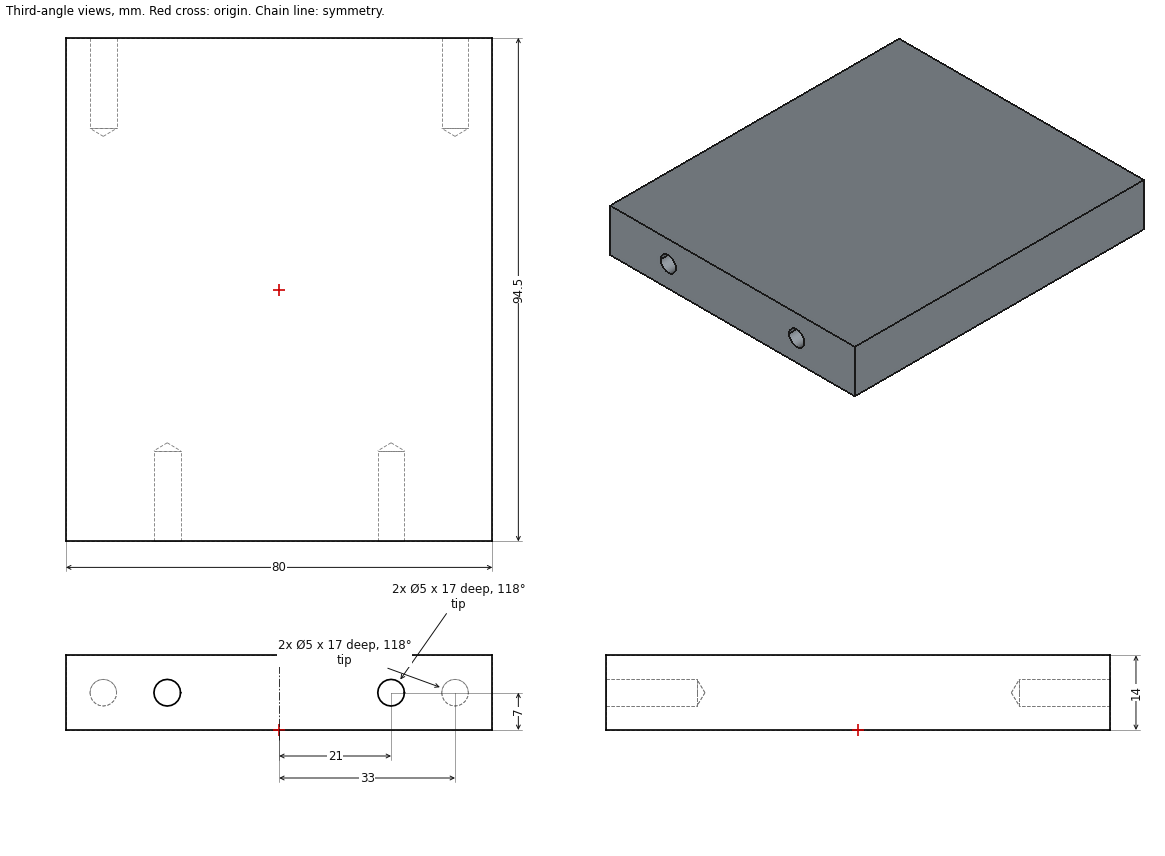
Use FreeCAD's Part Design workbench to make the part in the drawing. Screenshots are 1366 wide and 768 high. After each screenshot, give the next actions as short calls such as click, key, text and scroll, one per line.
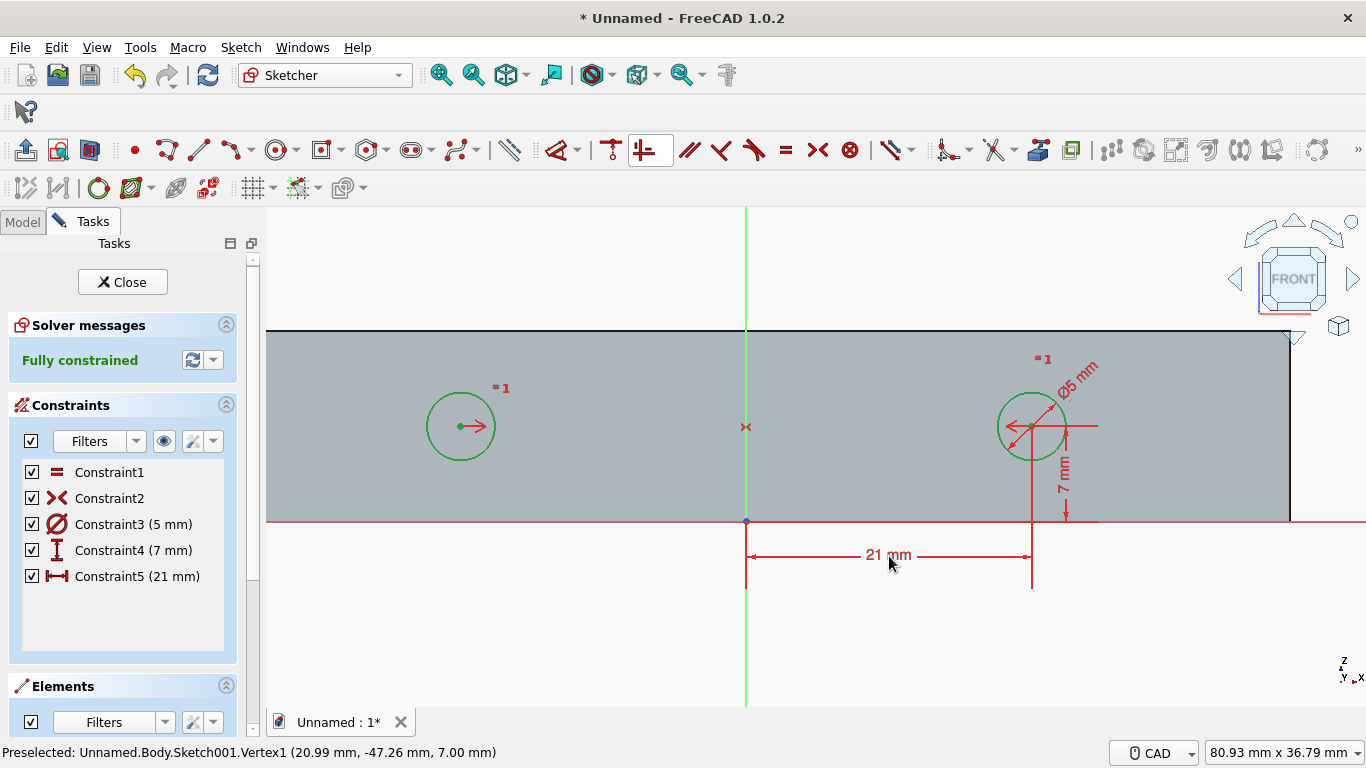
click(123, 282)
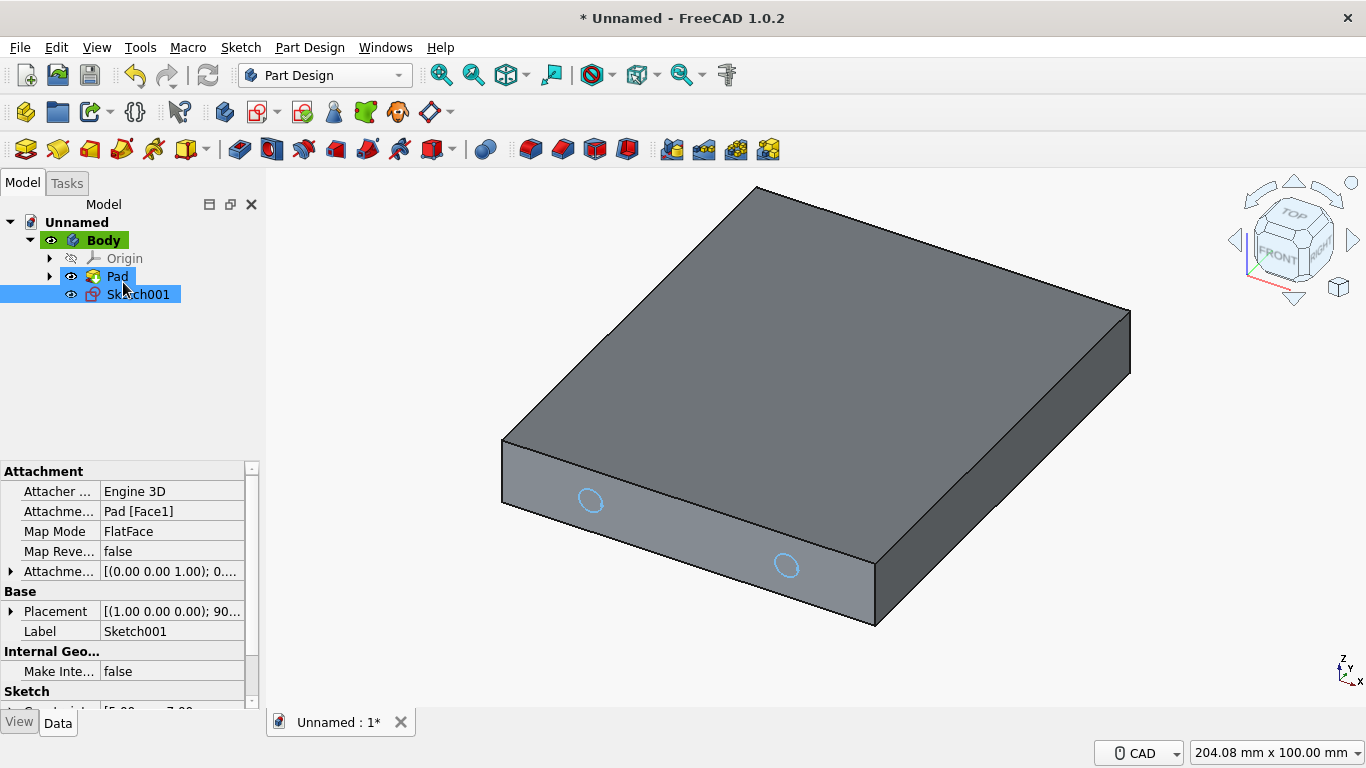
click(272, 150)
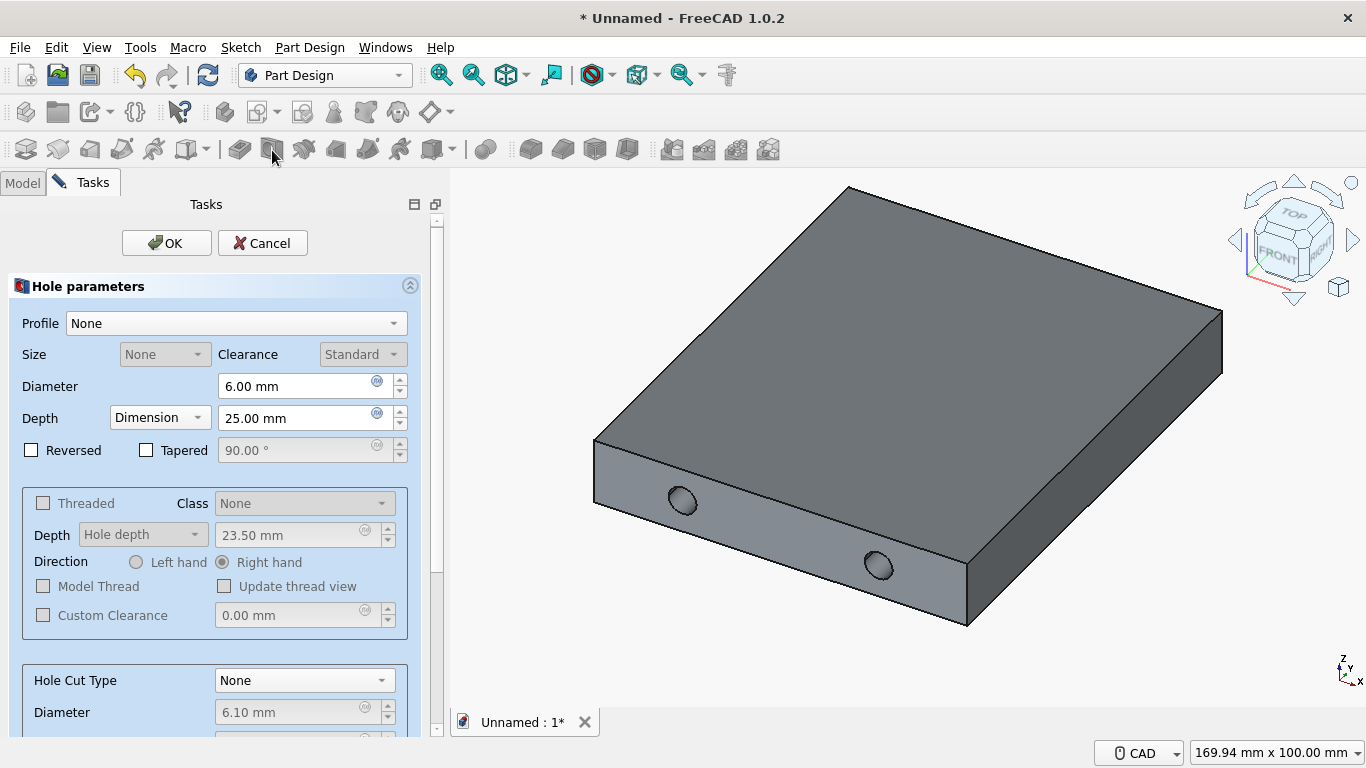
triple_click(305, 386)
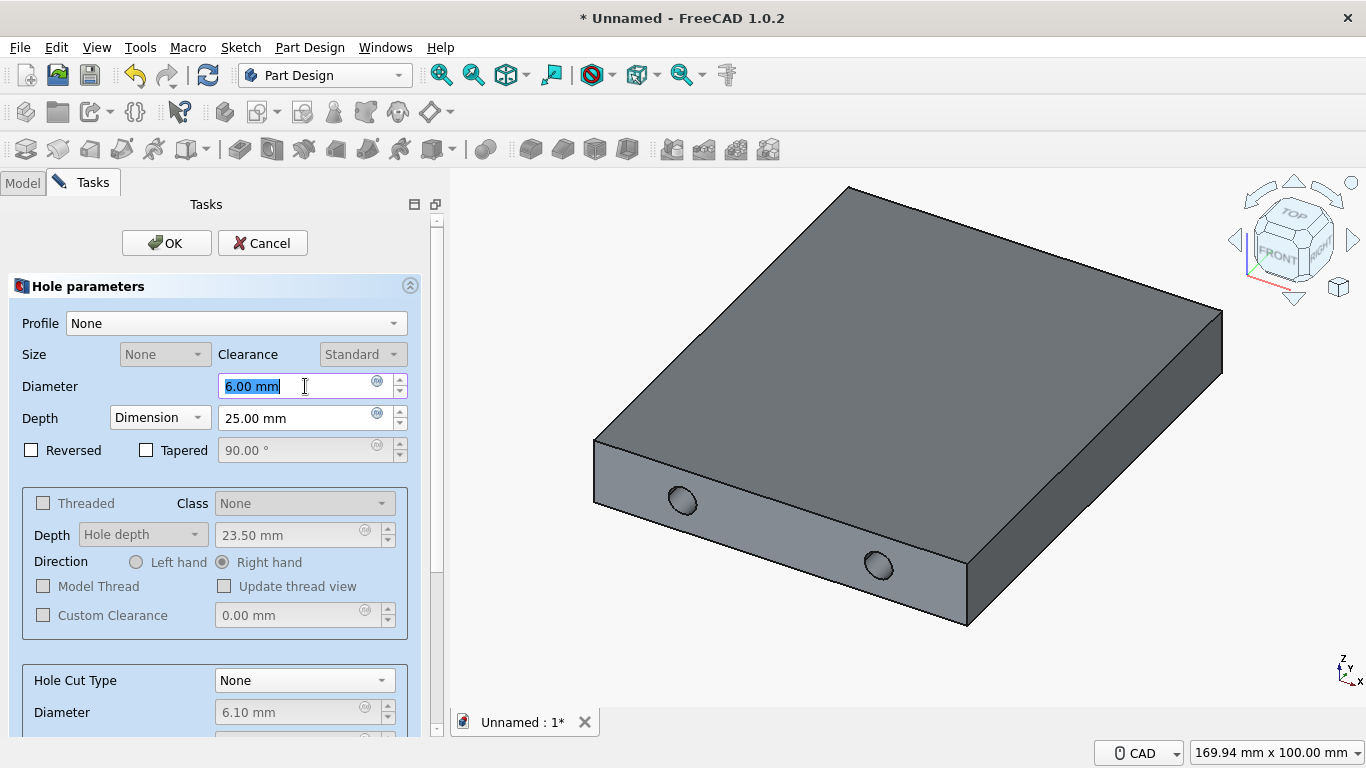
text(5)
key(Tab)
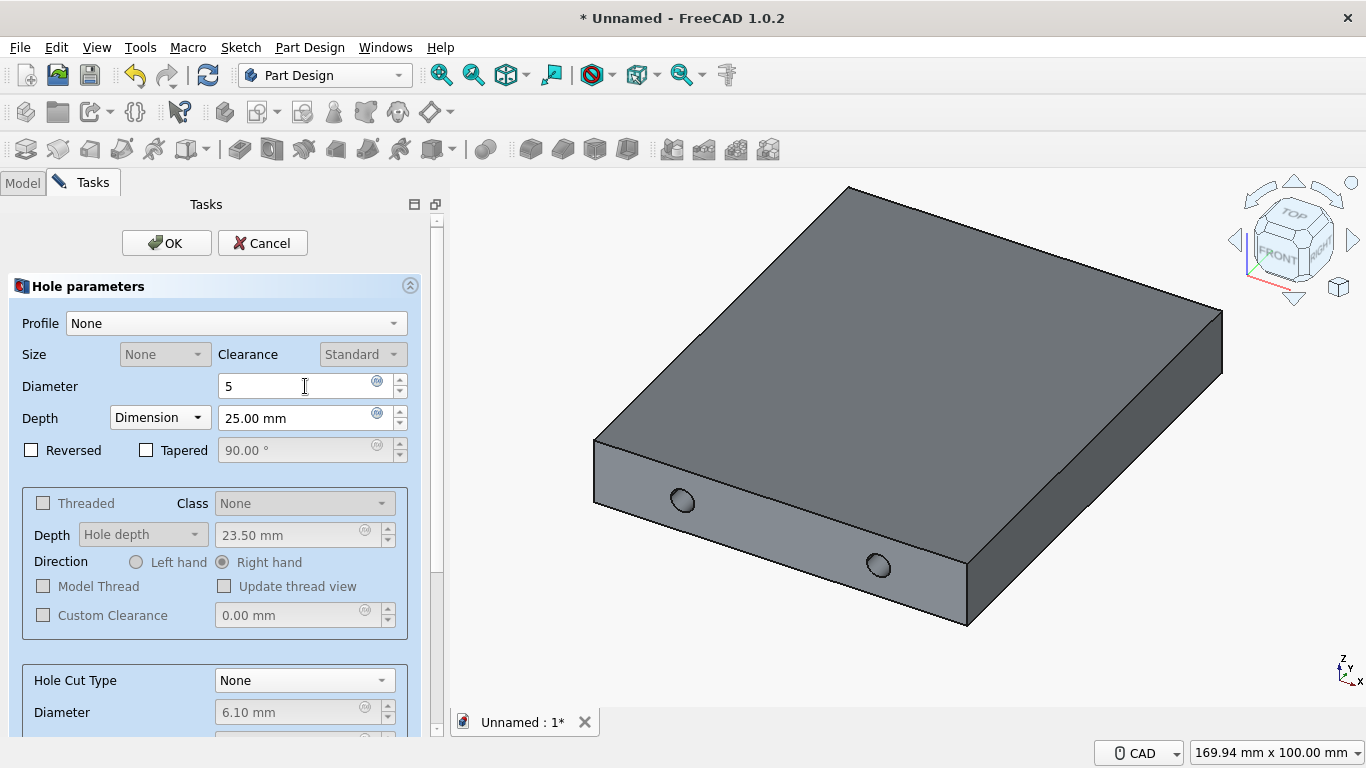
triple_click(305, 418)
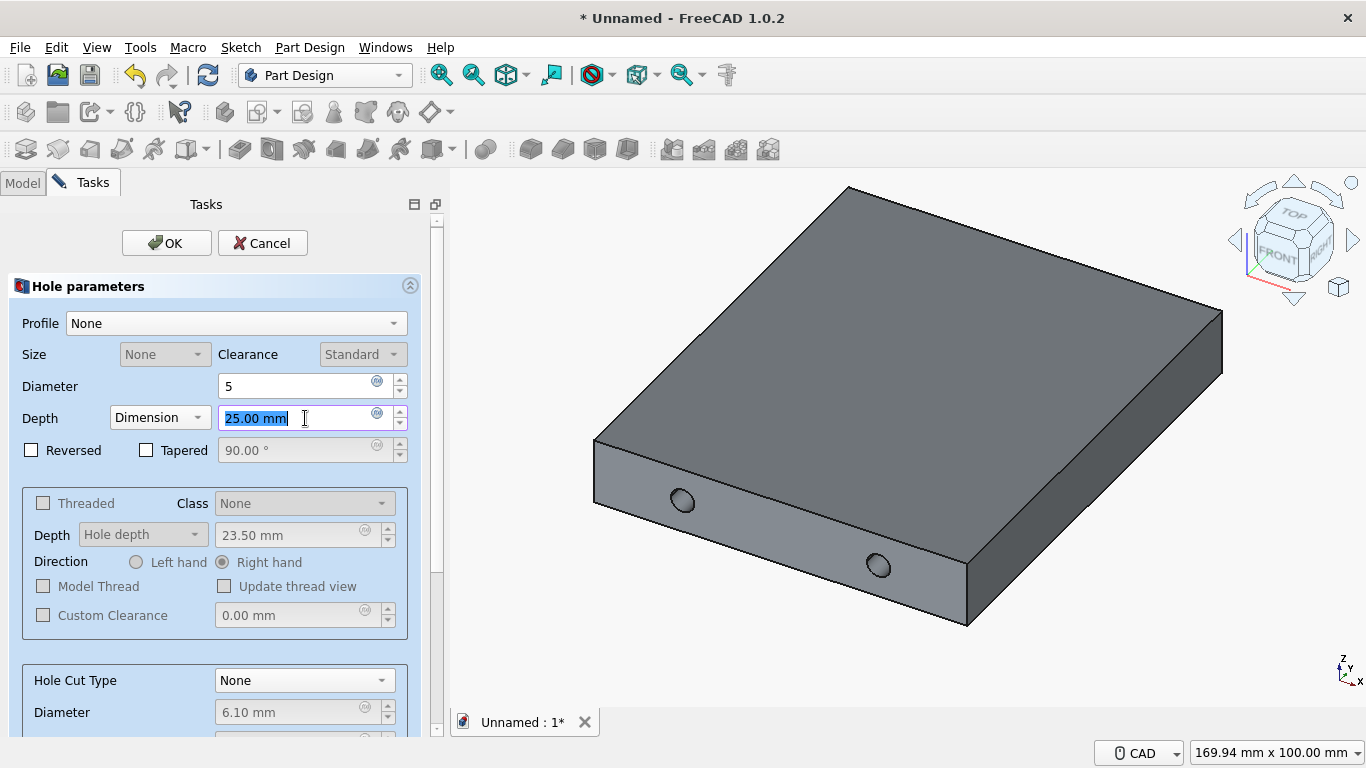
text(17)
key(Tab)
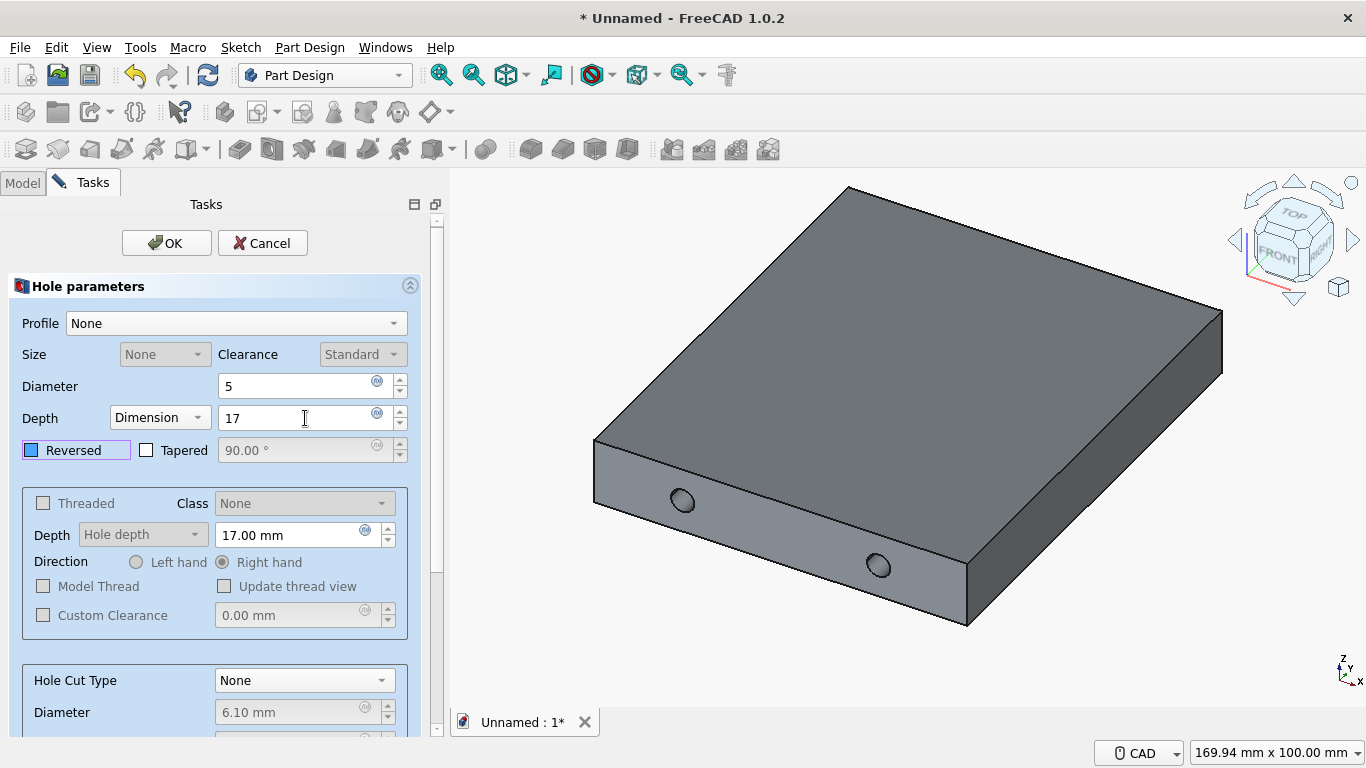
click(167, 243)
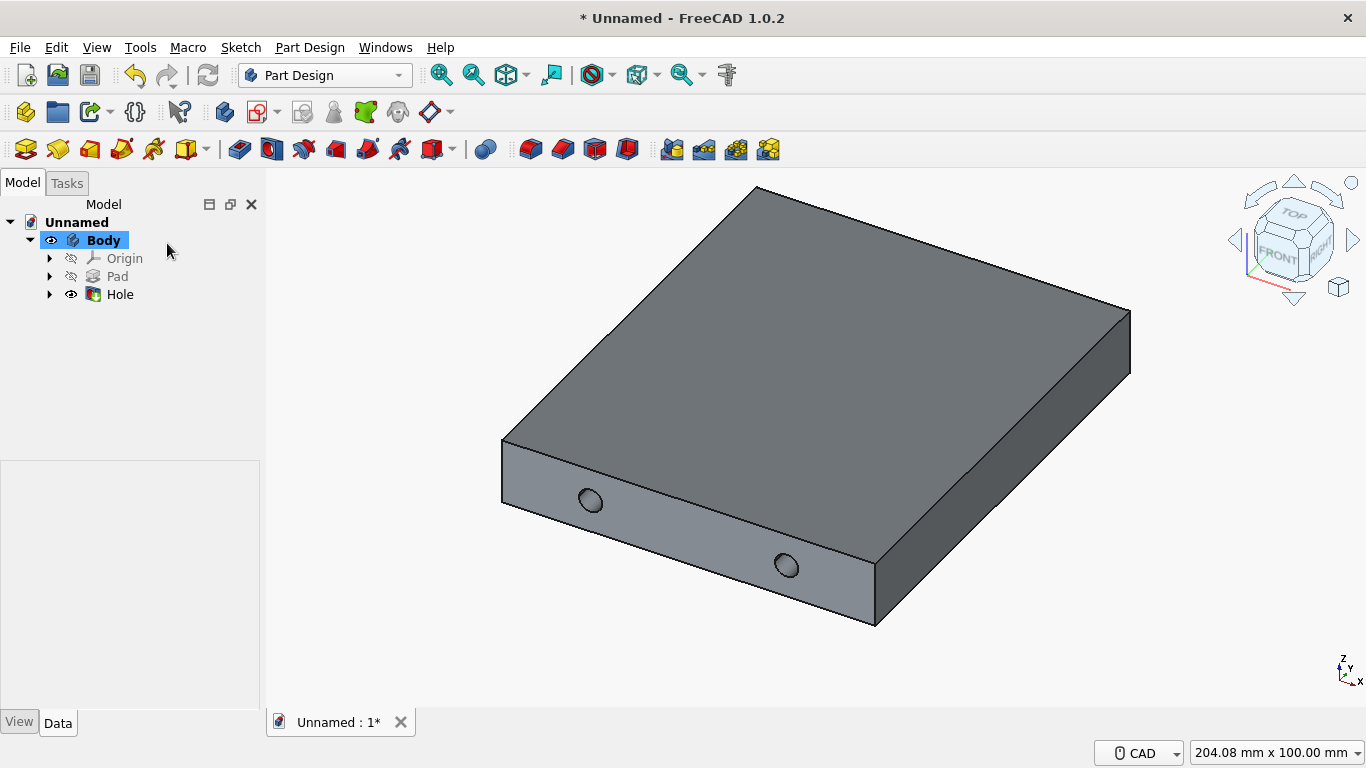
key(4)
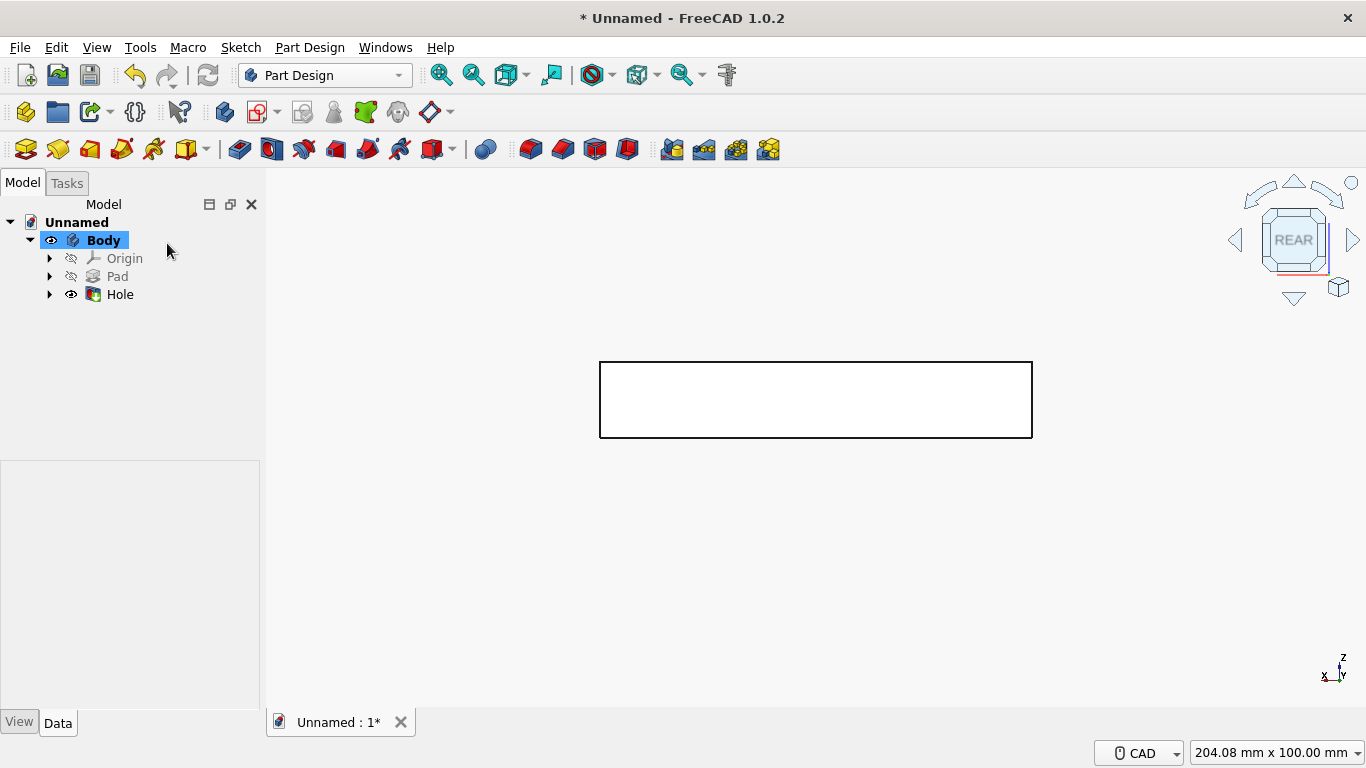
click(442, 76)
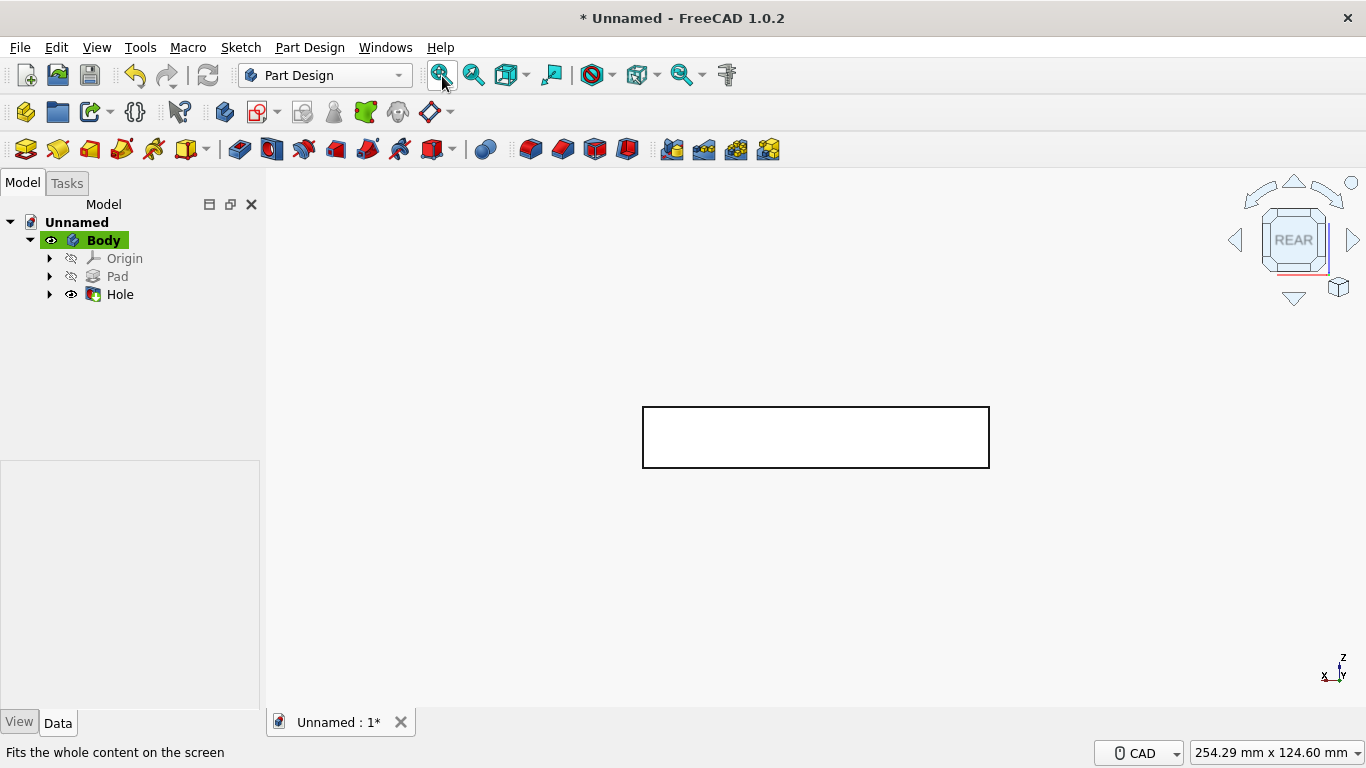
click(717, 437)